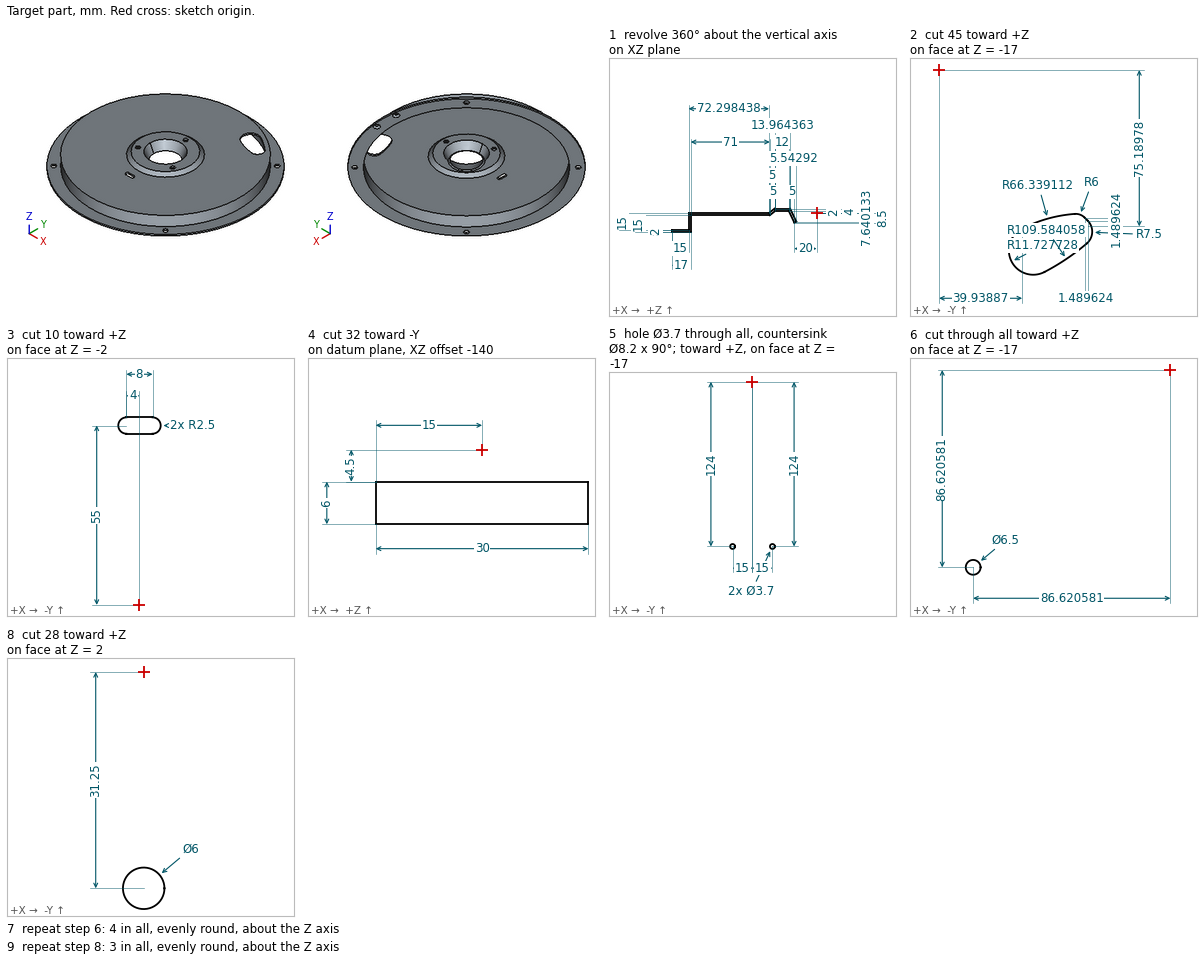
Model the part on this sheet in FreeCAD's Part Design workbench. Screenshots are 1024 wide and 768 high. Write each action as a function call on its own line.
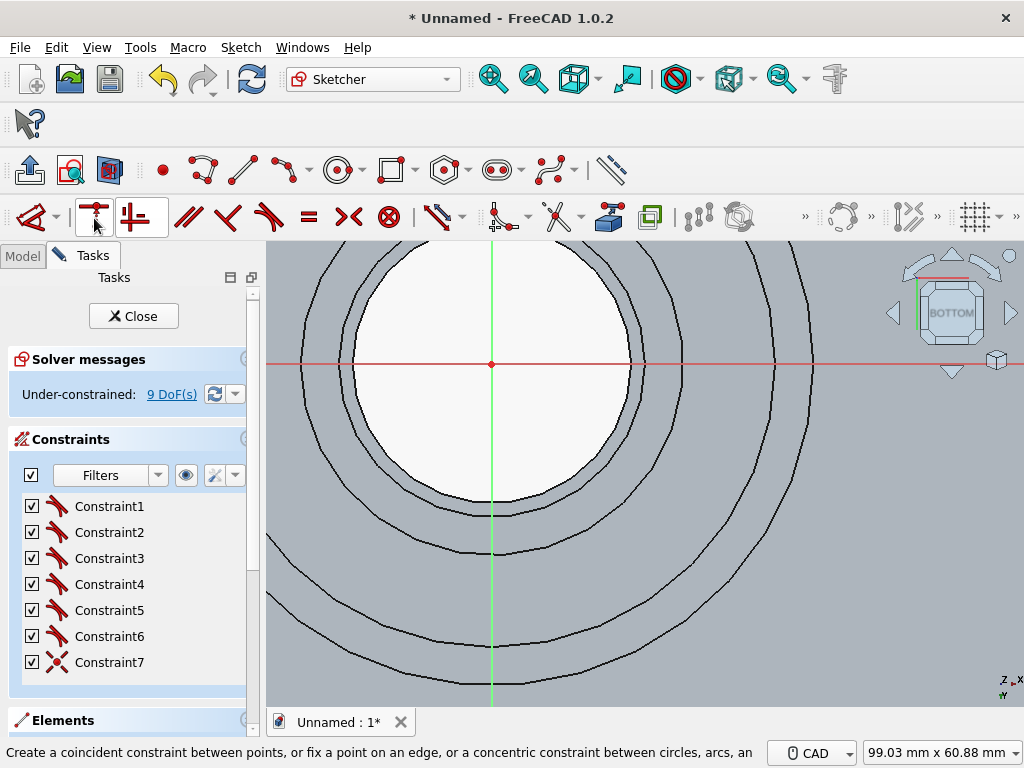
key(d)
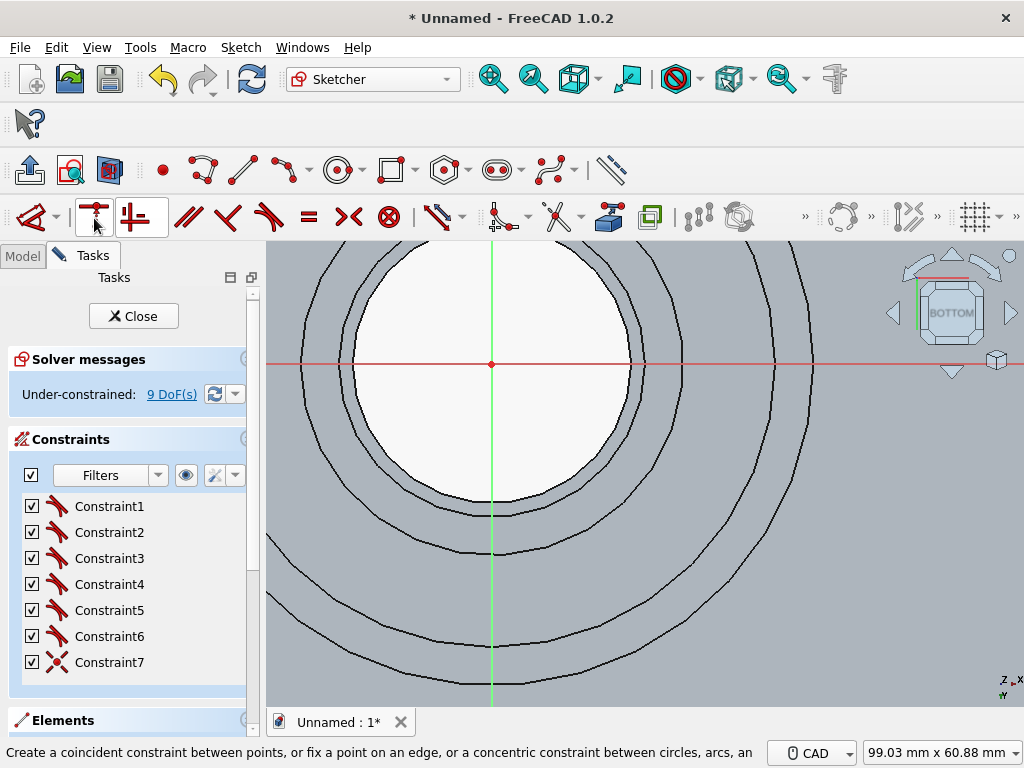
scroll(576, 474, down, 5)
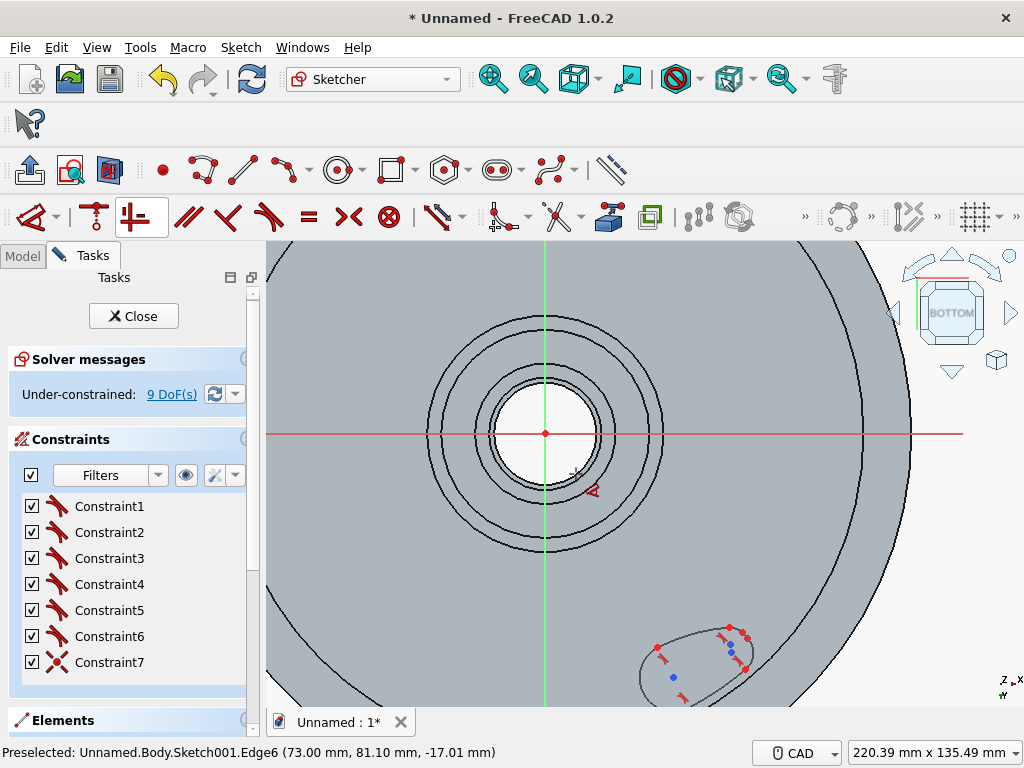
scroll(576, 474, down, 5)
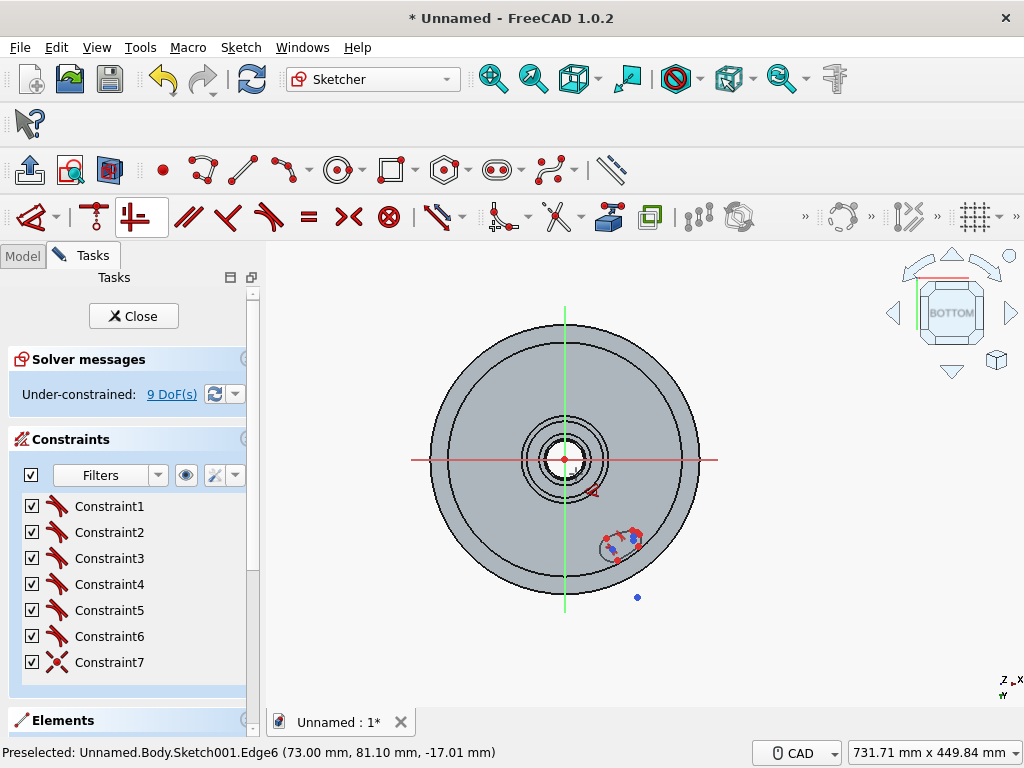
scroll(627, 555, up, 11)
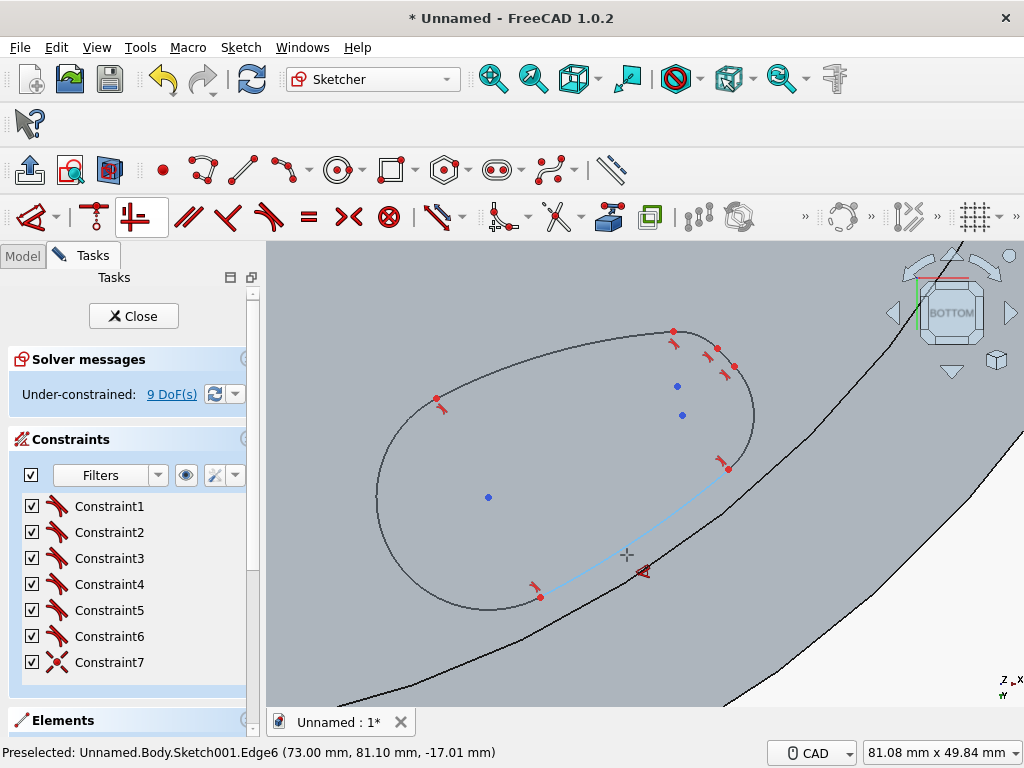
click(706, 340)
click(723, 313)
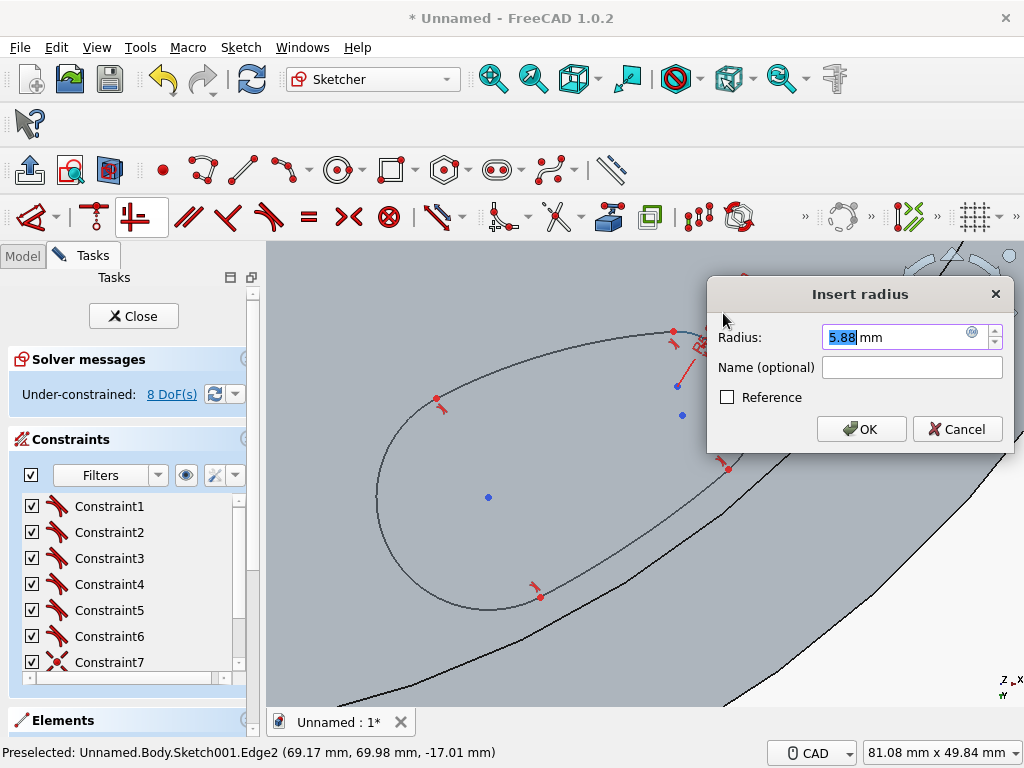
text(6)
key(Return)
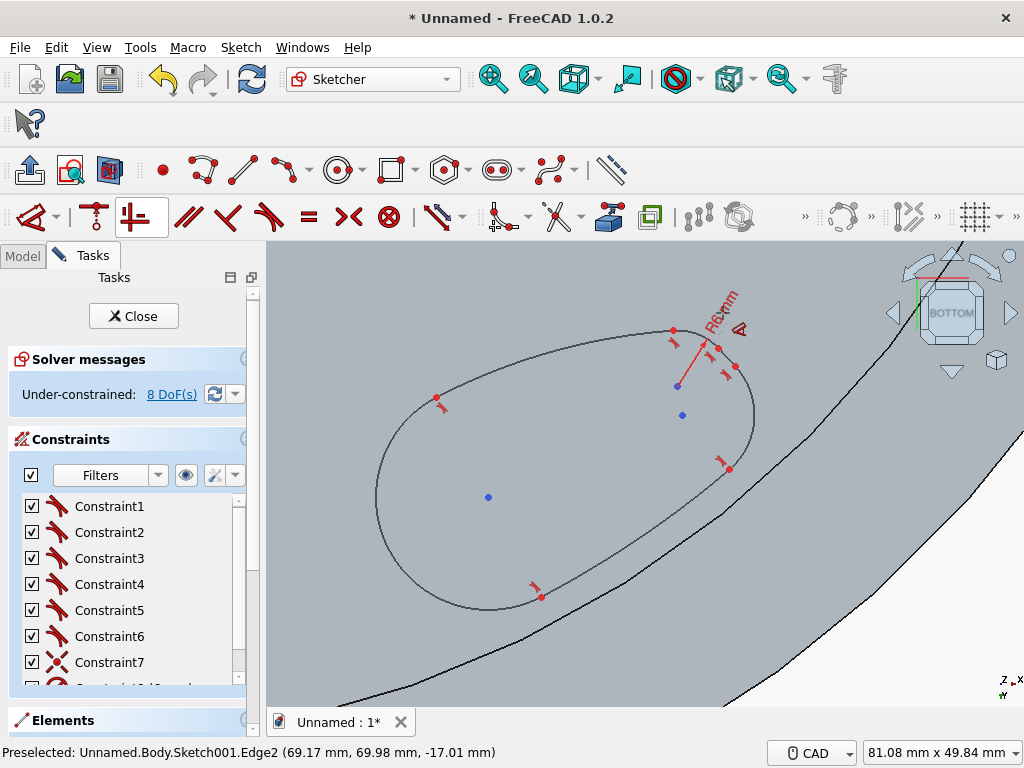
click(600, 340)
click(594, 309)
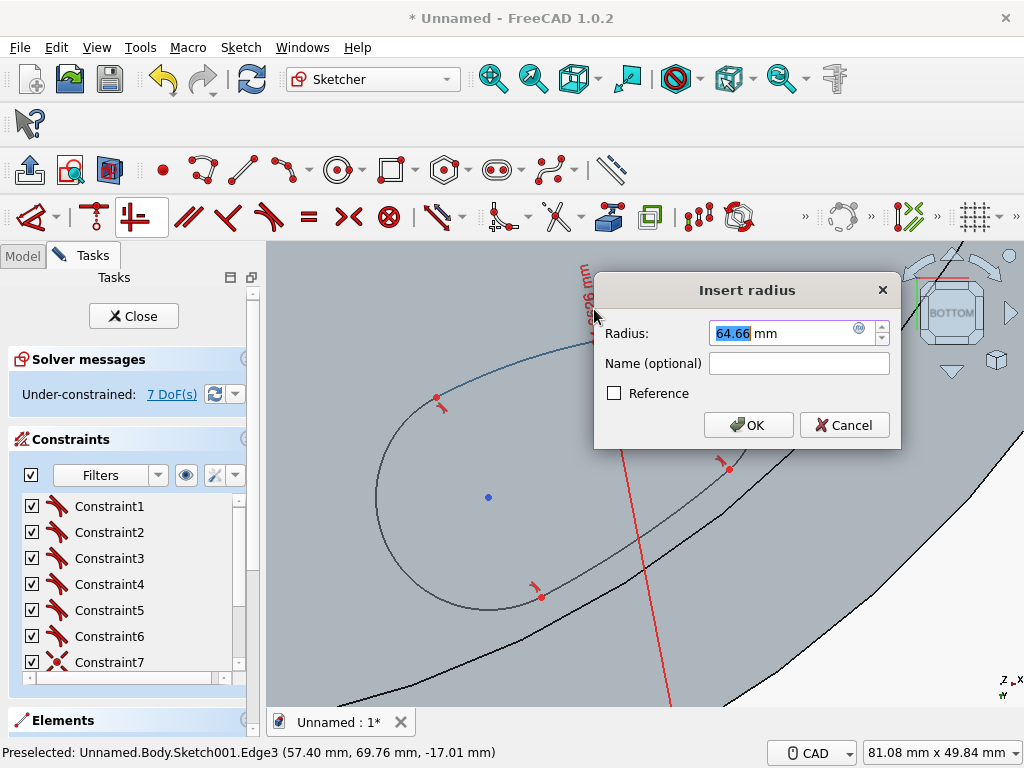
text(66.339112)
key(Return)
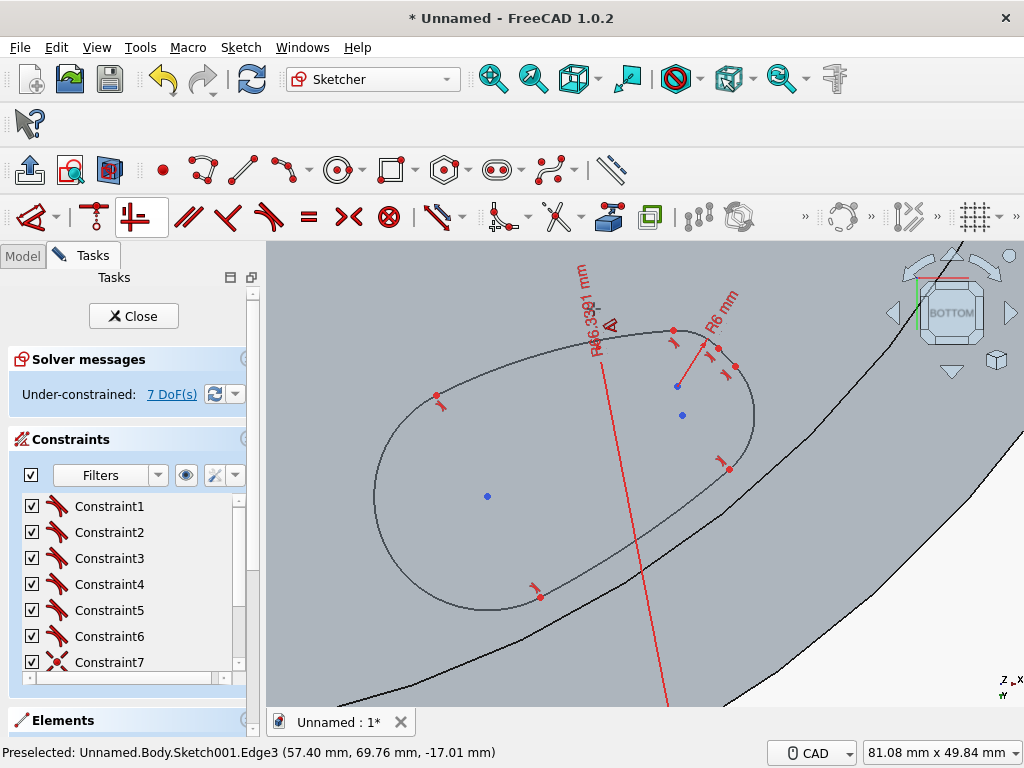
click(376, 479)
click(344, 474)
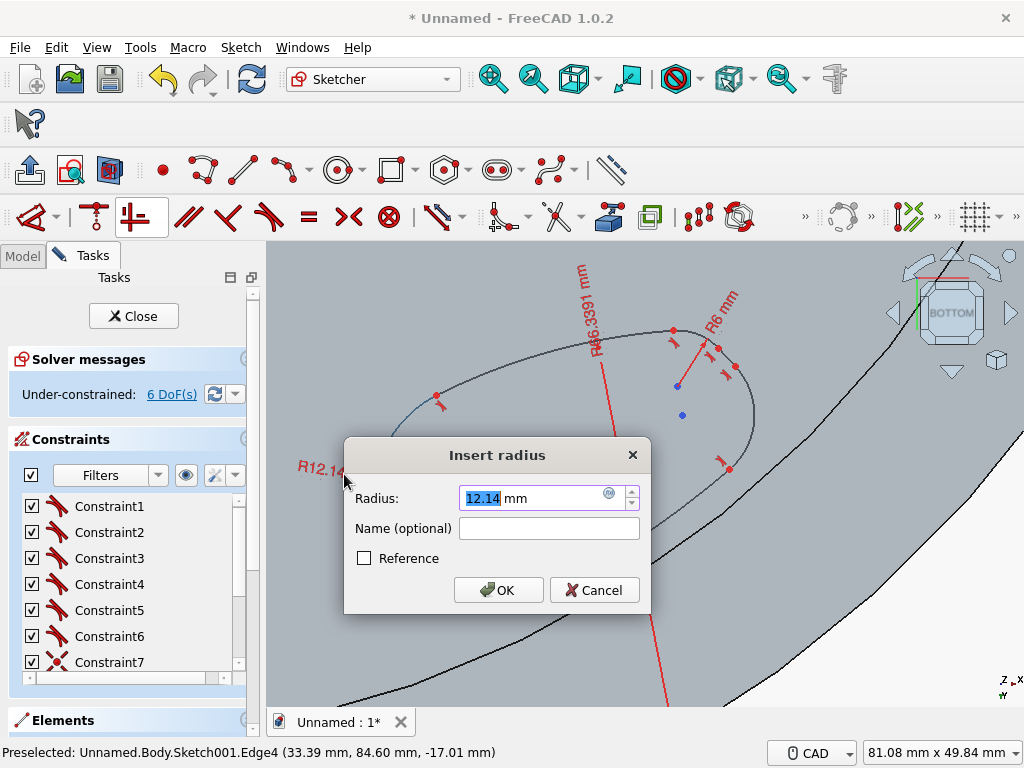
text(11.727728)
key(Return)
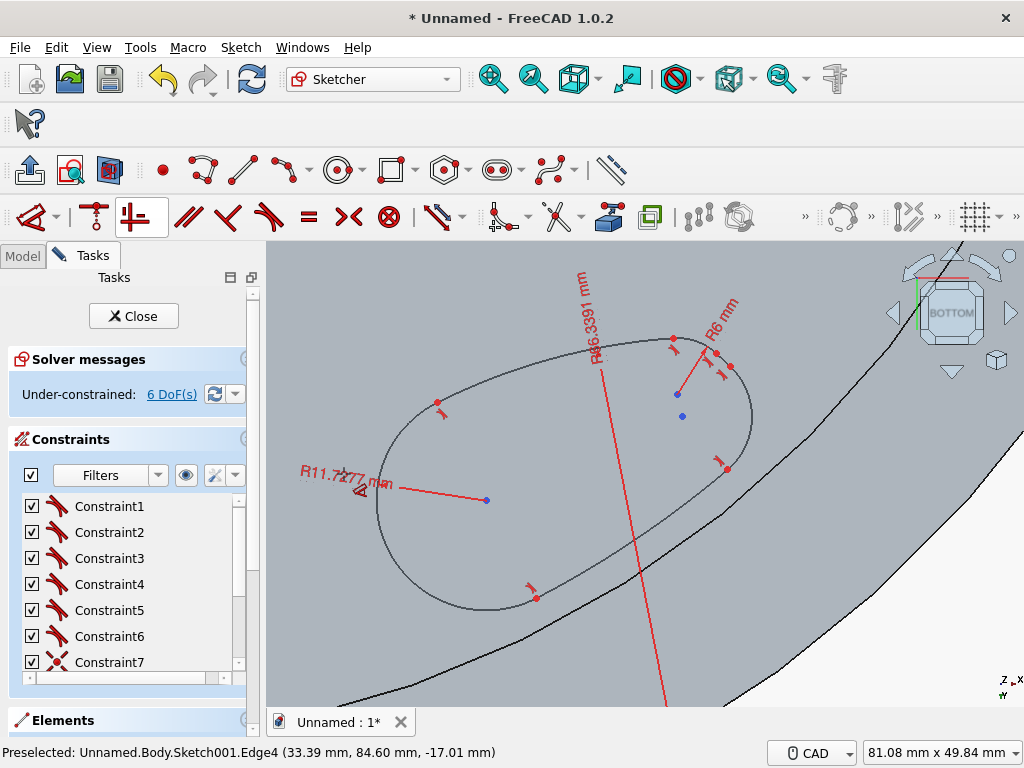
click(597, 564)
click(614, 591)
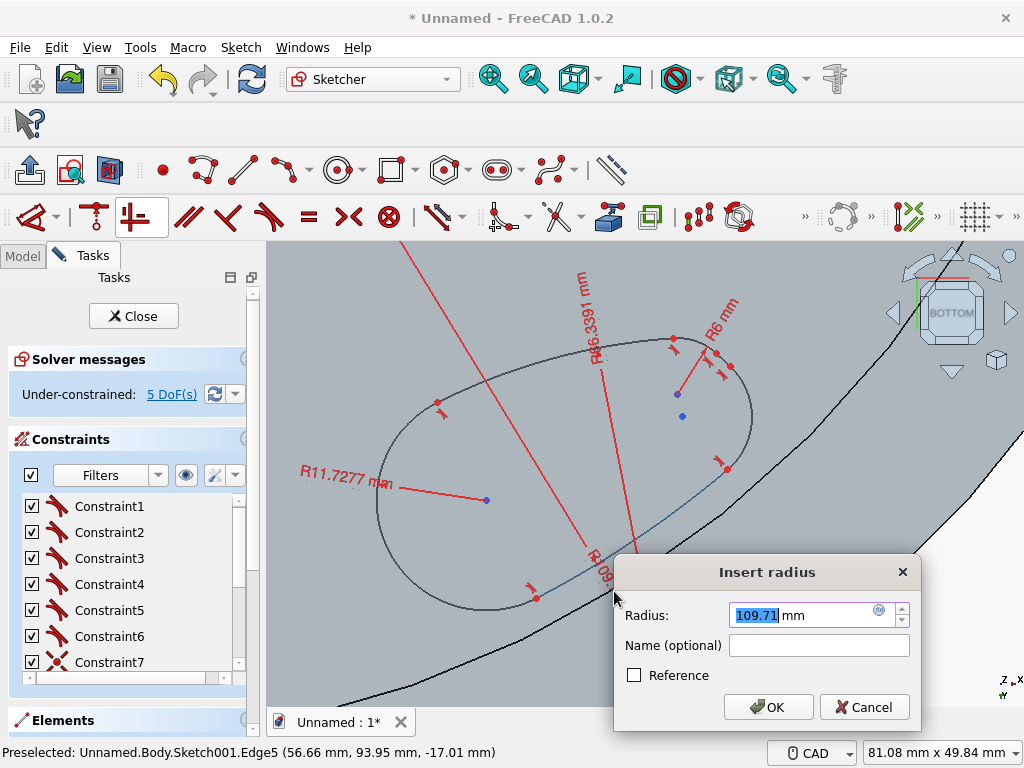
text(109.584058)
key(Return)